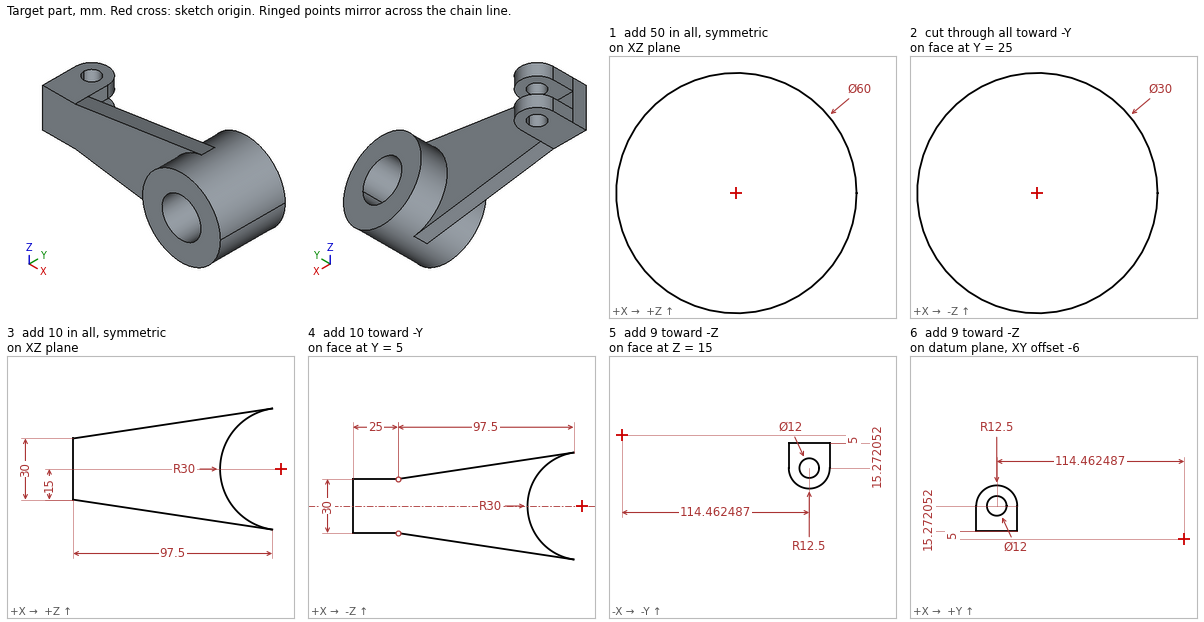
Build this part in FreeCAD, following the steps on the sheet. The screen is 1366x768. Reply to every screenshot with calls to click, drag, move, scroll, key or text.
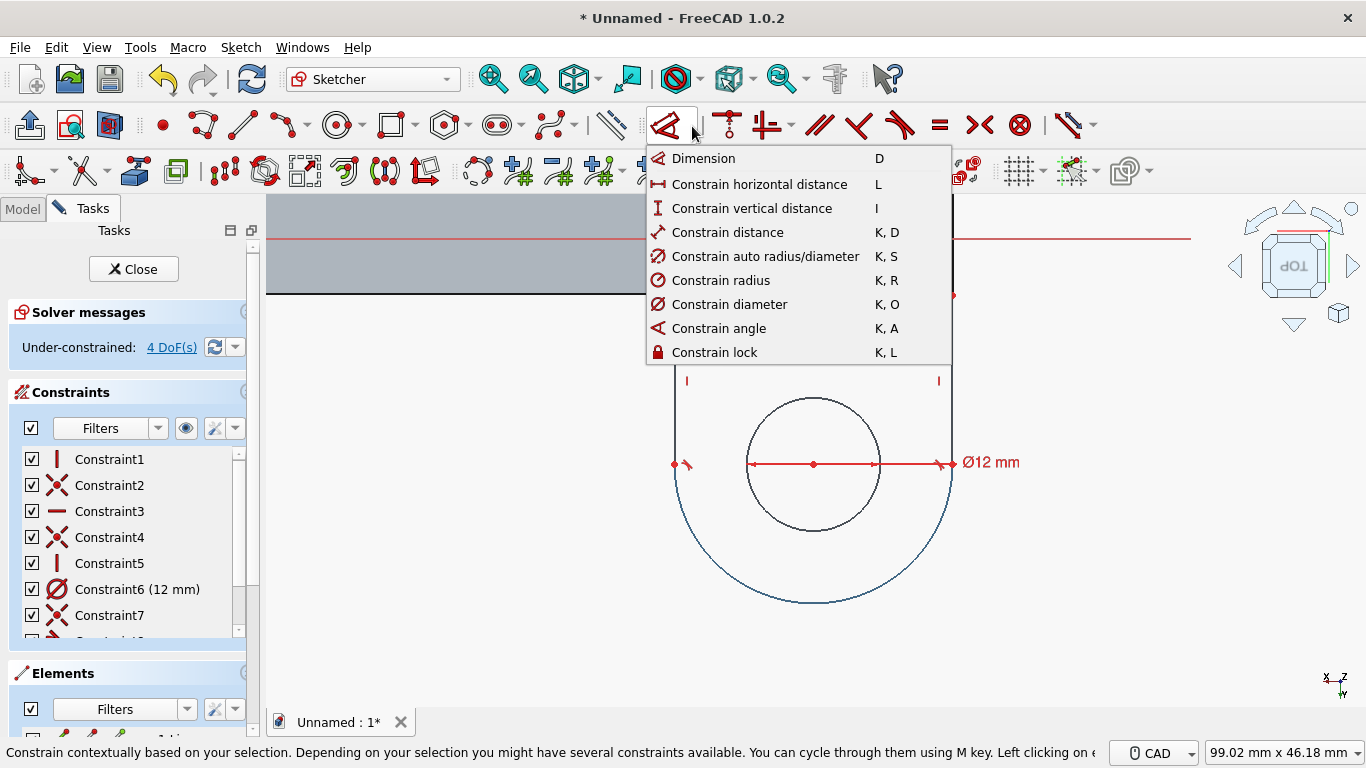
click(799, 280)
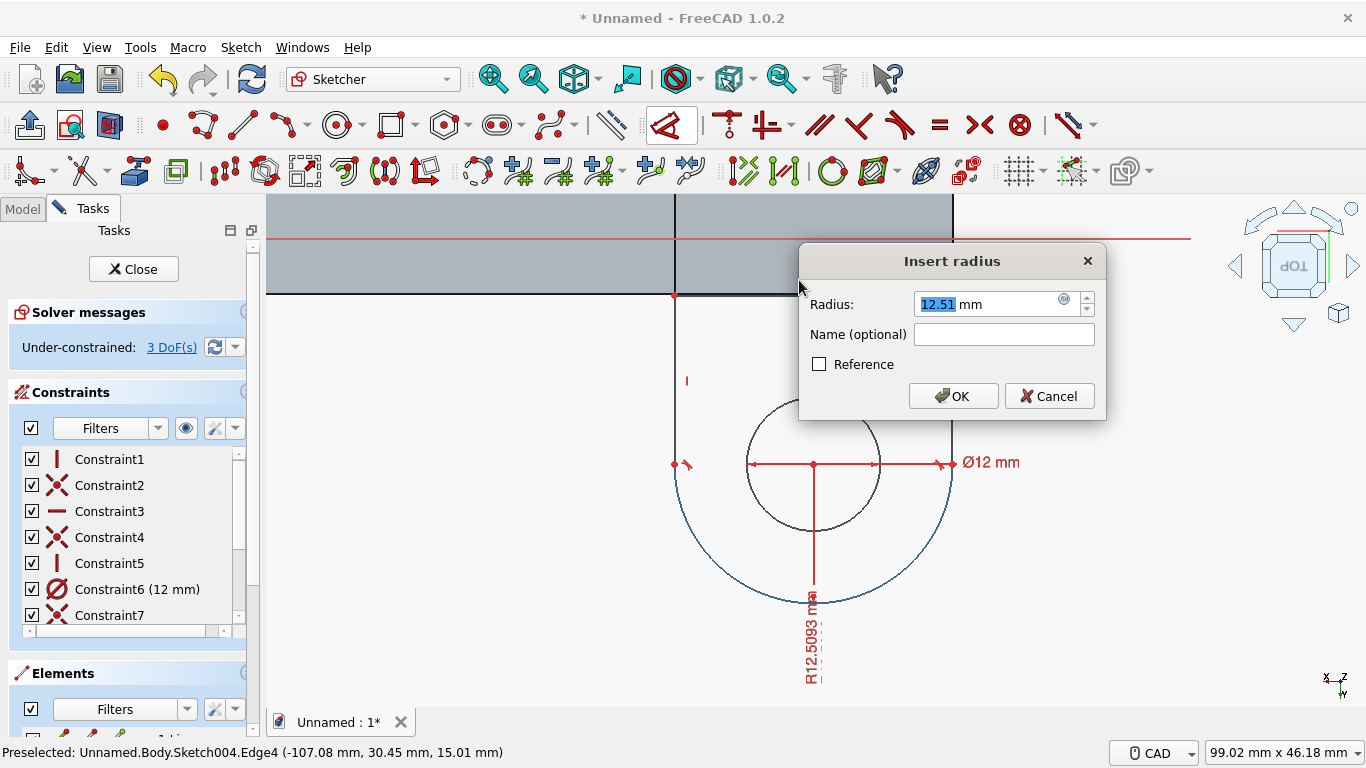
text(12.5)
key(Return)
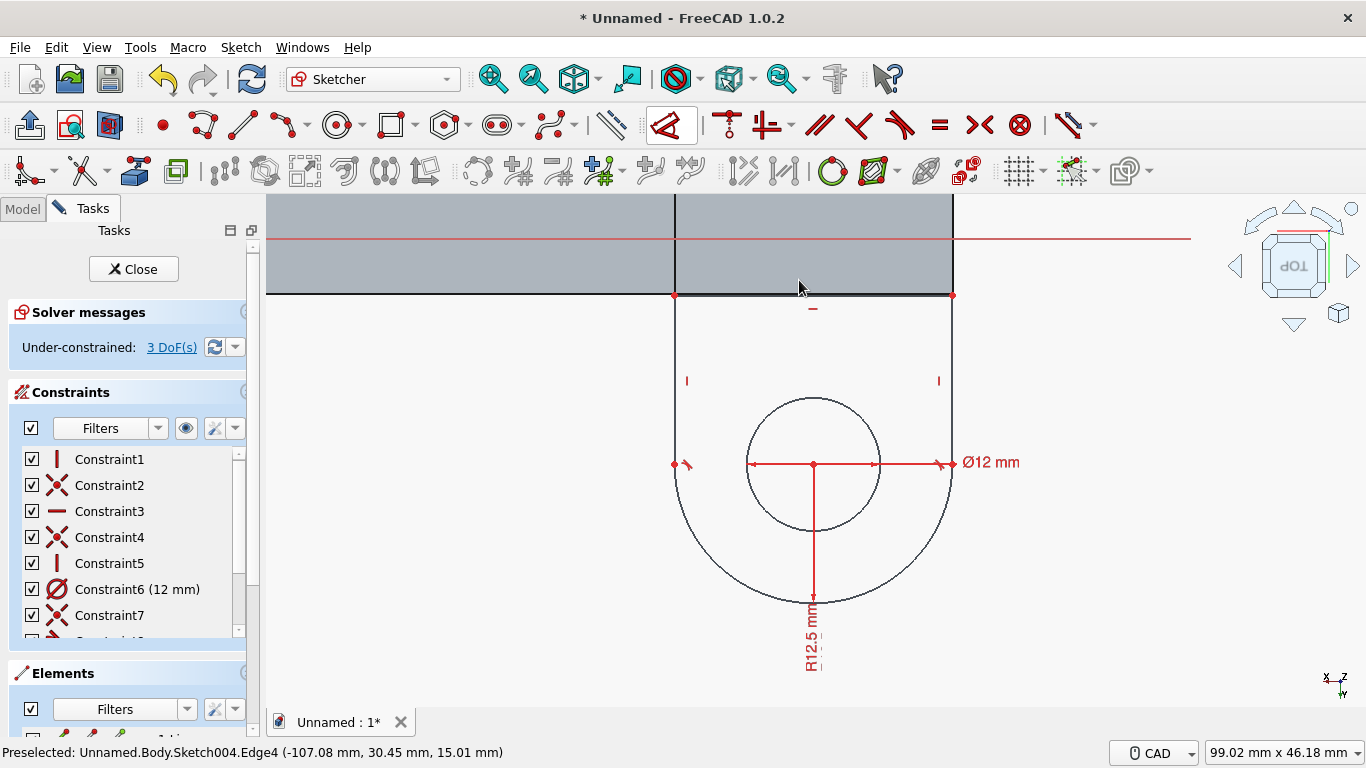
click(952, 296)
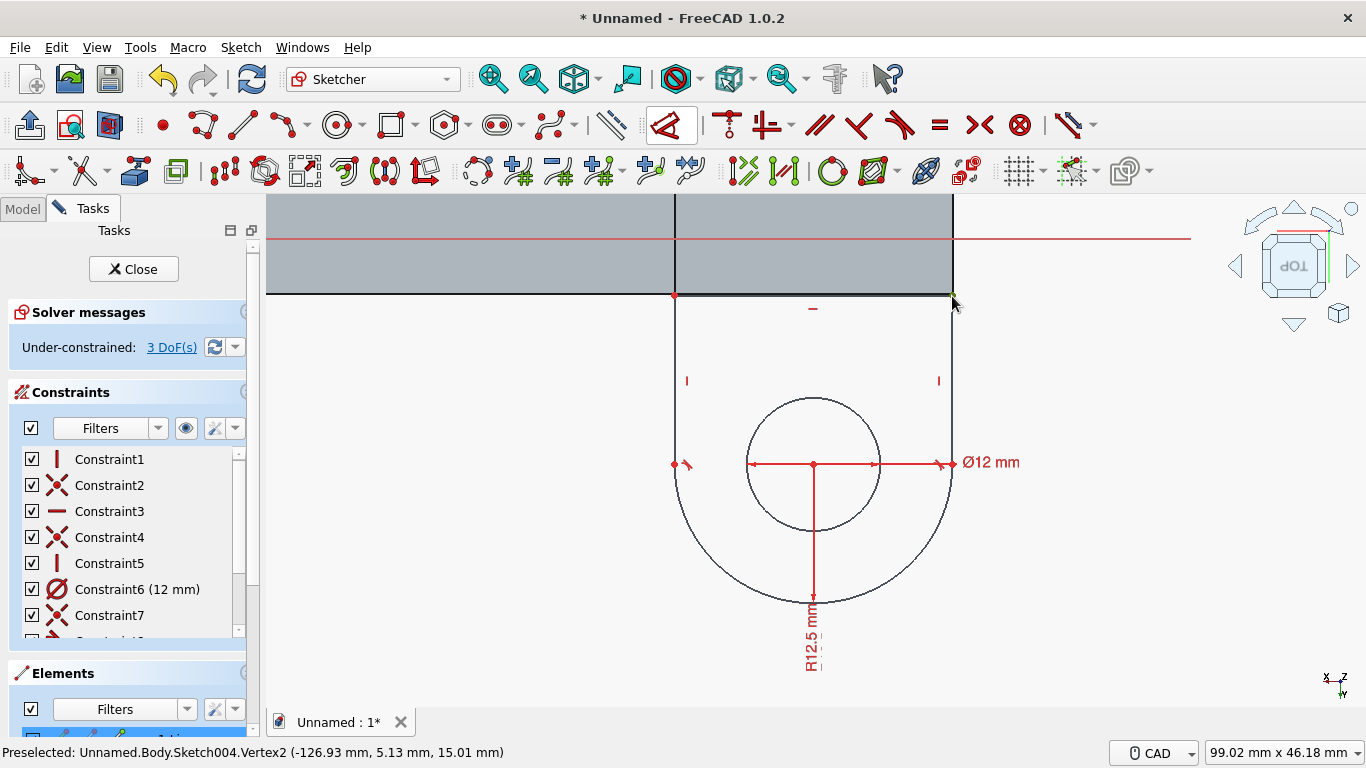
key(i)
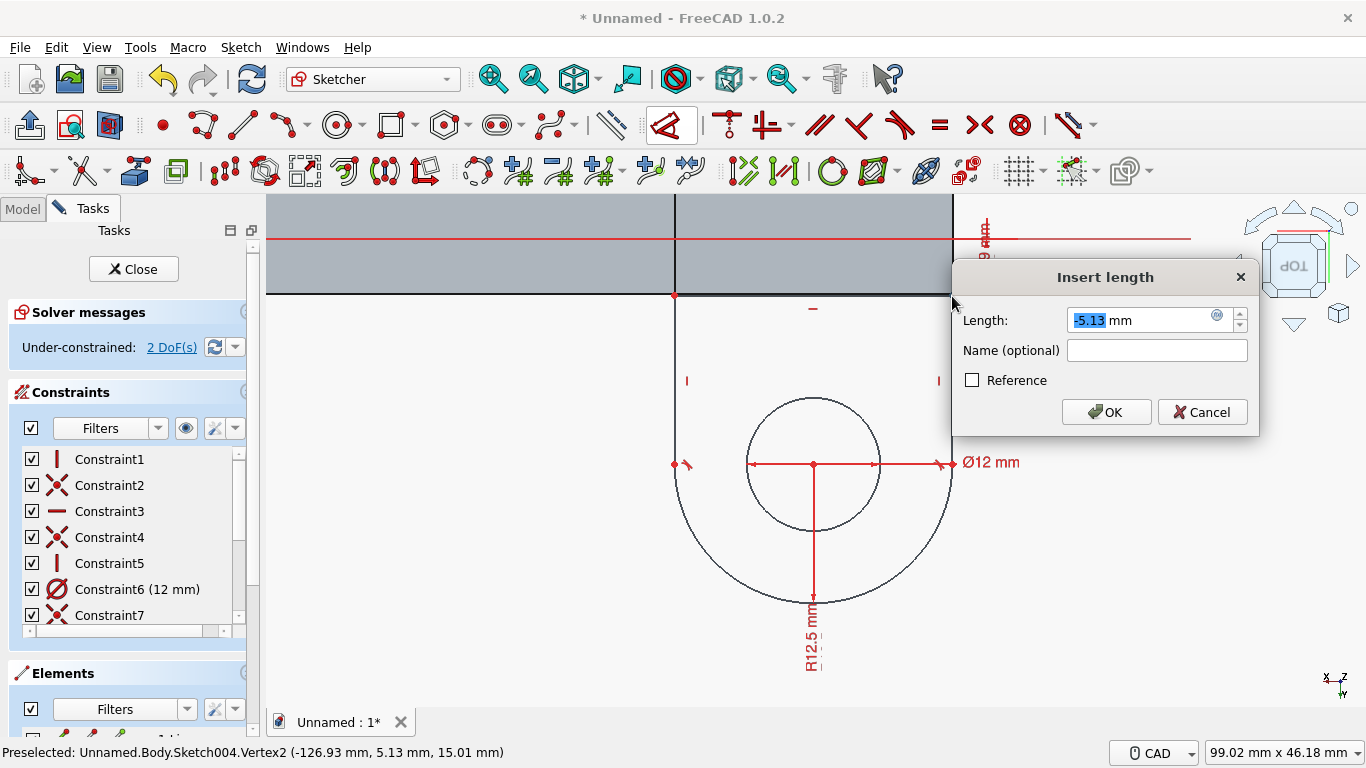
text(-5)
key(Return)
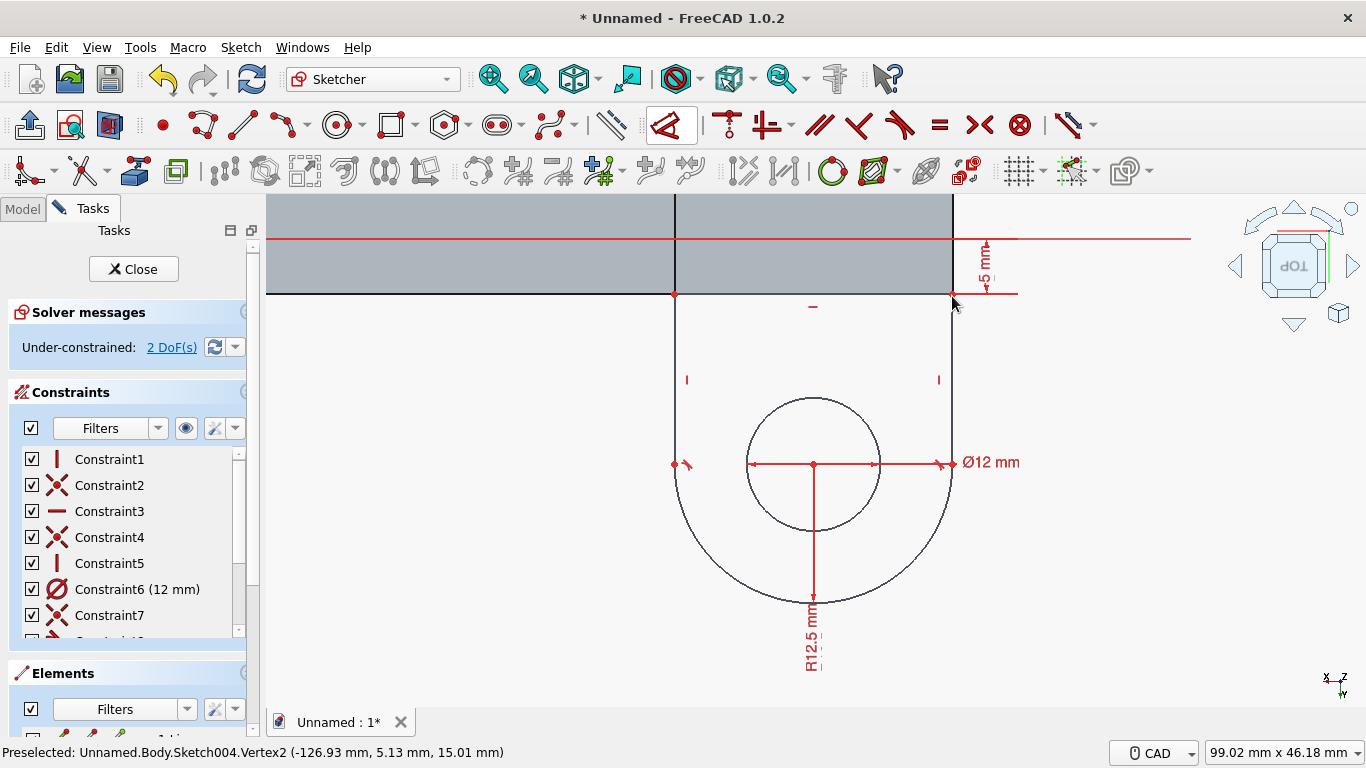
click(952, 413)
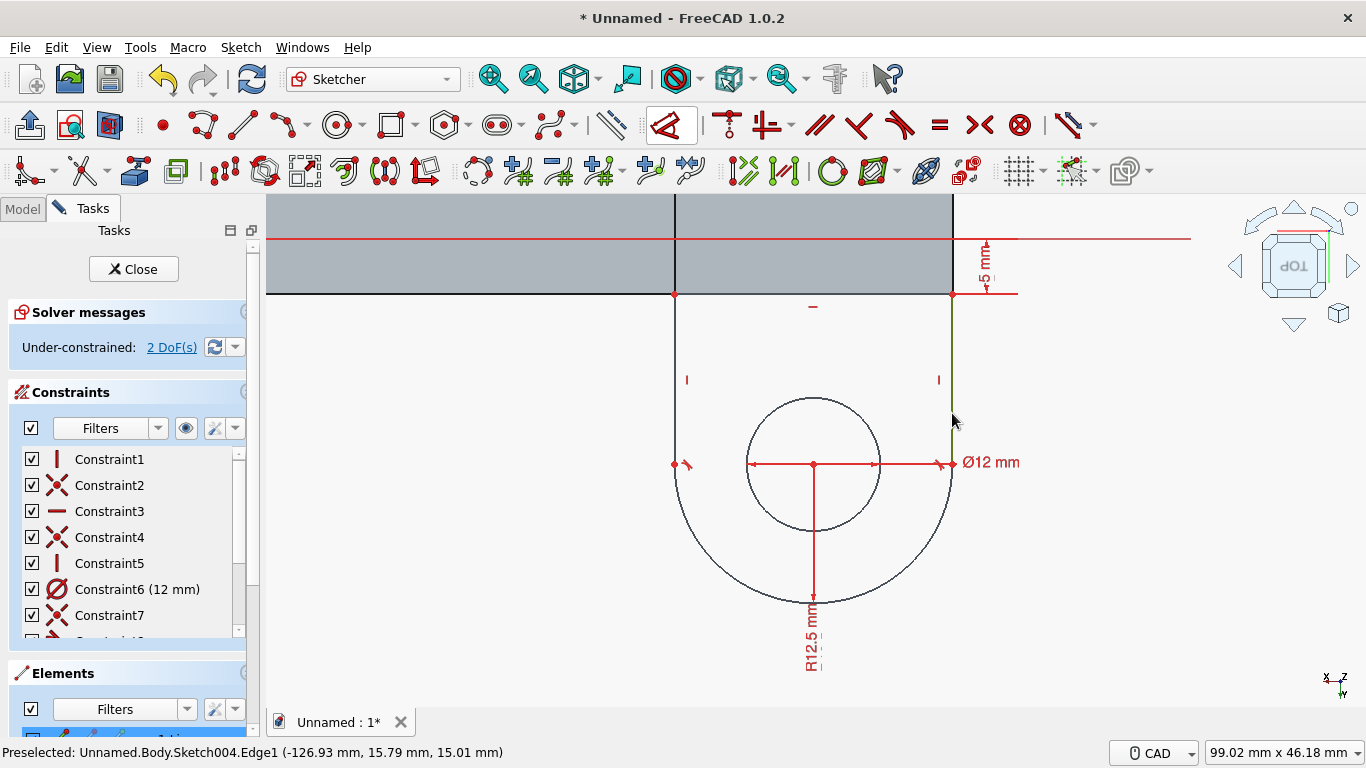
key(i)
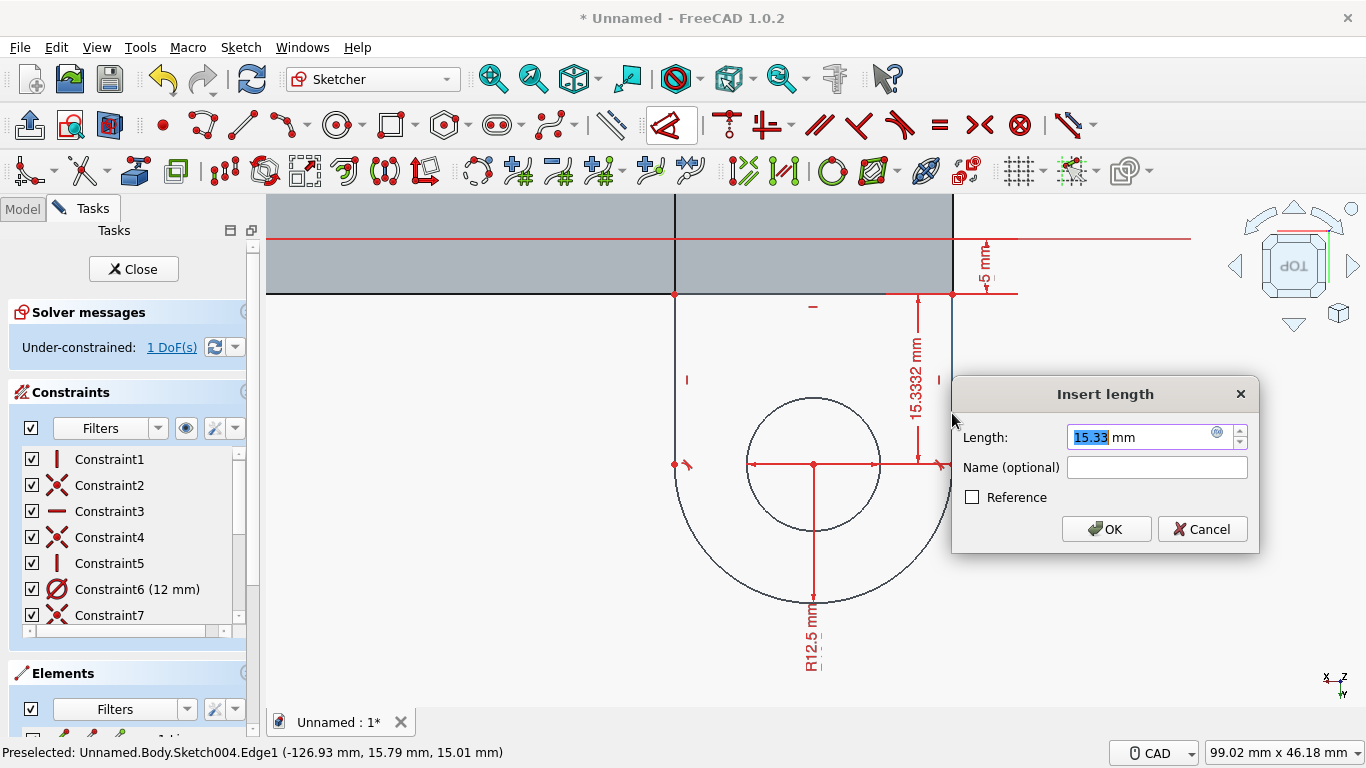
text(15.272052)
key(Return)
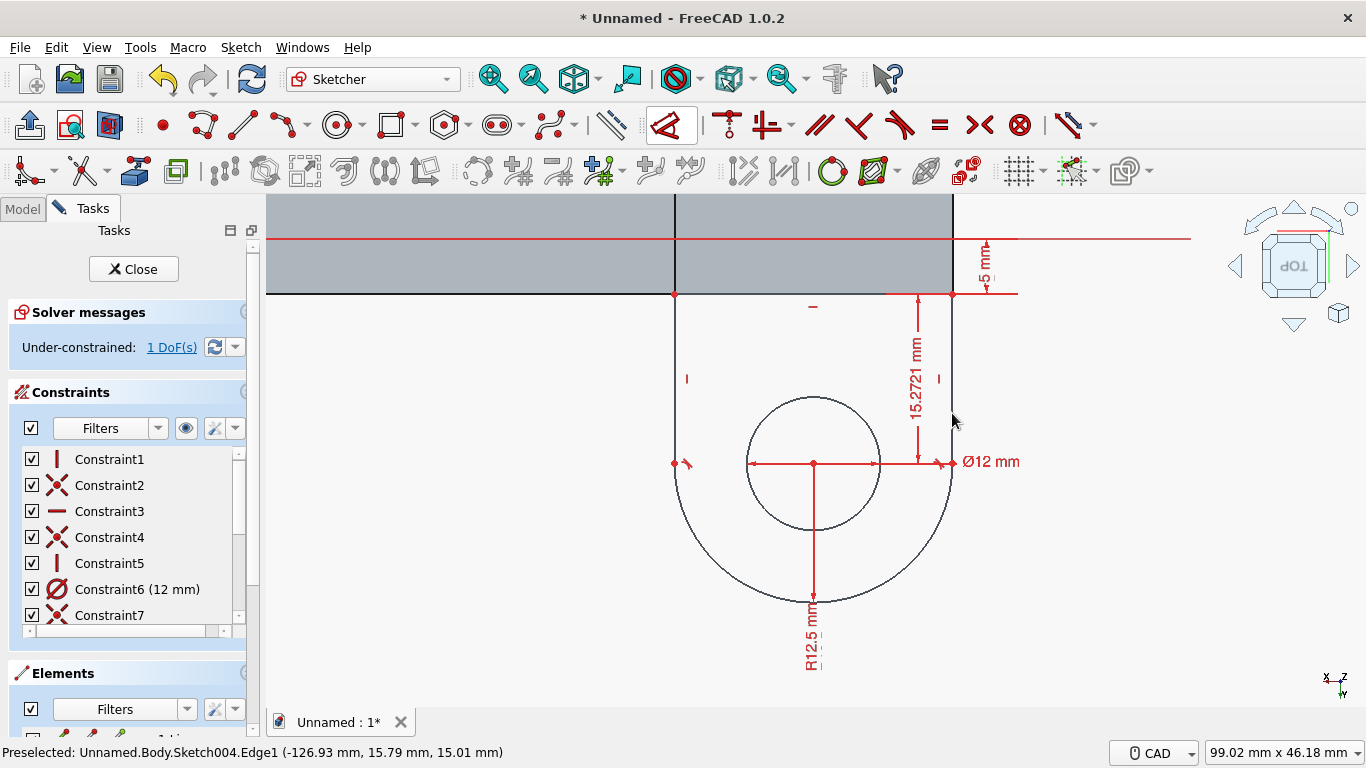
click(814, 464)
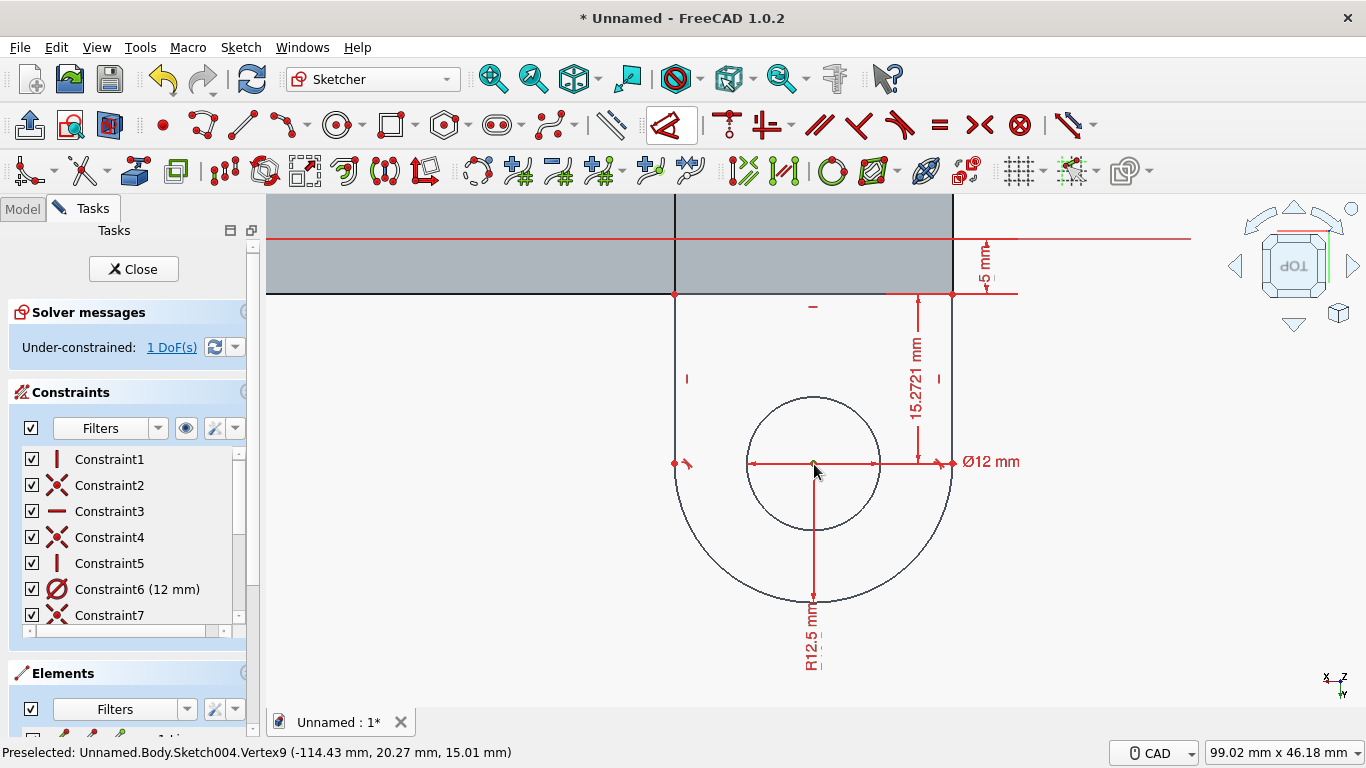
key(l)